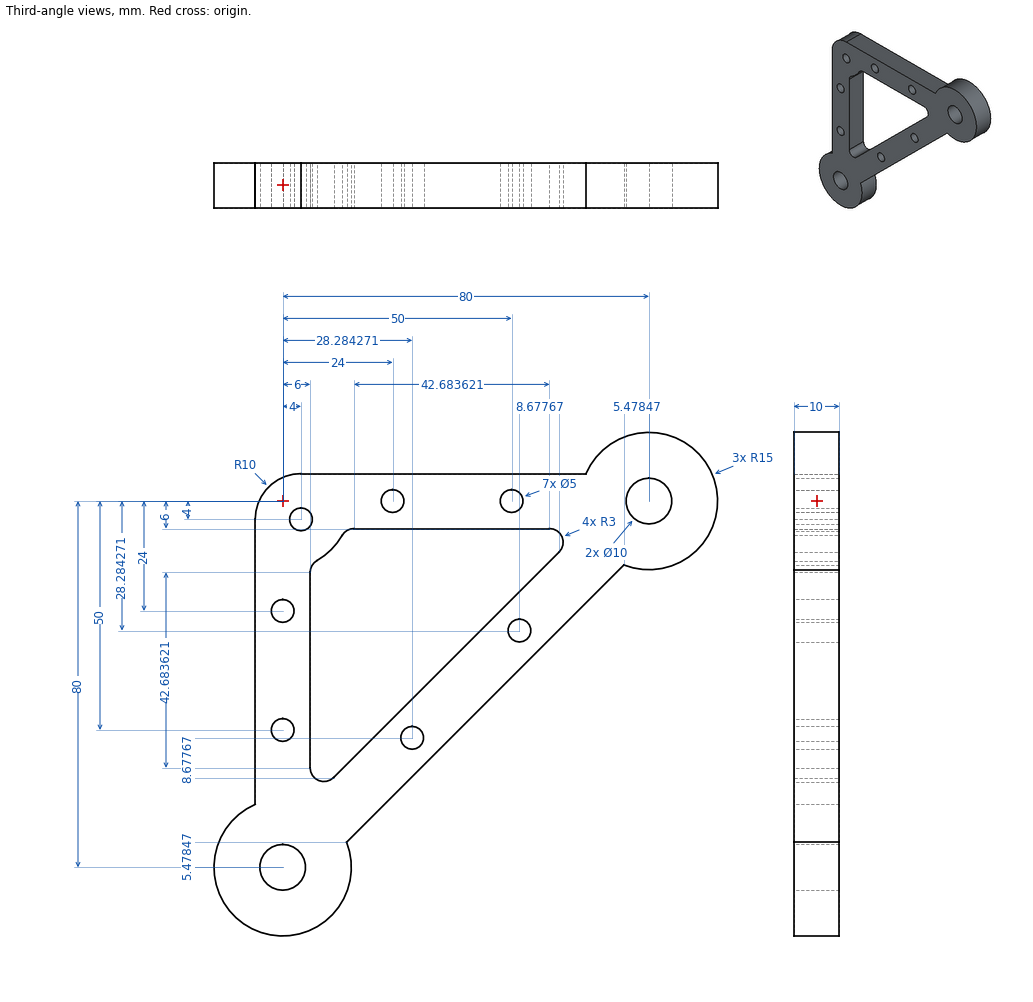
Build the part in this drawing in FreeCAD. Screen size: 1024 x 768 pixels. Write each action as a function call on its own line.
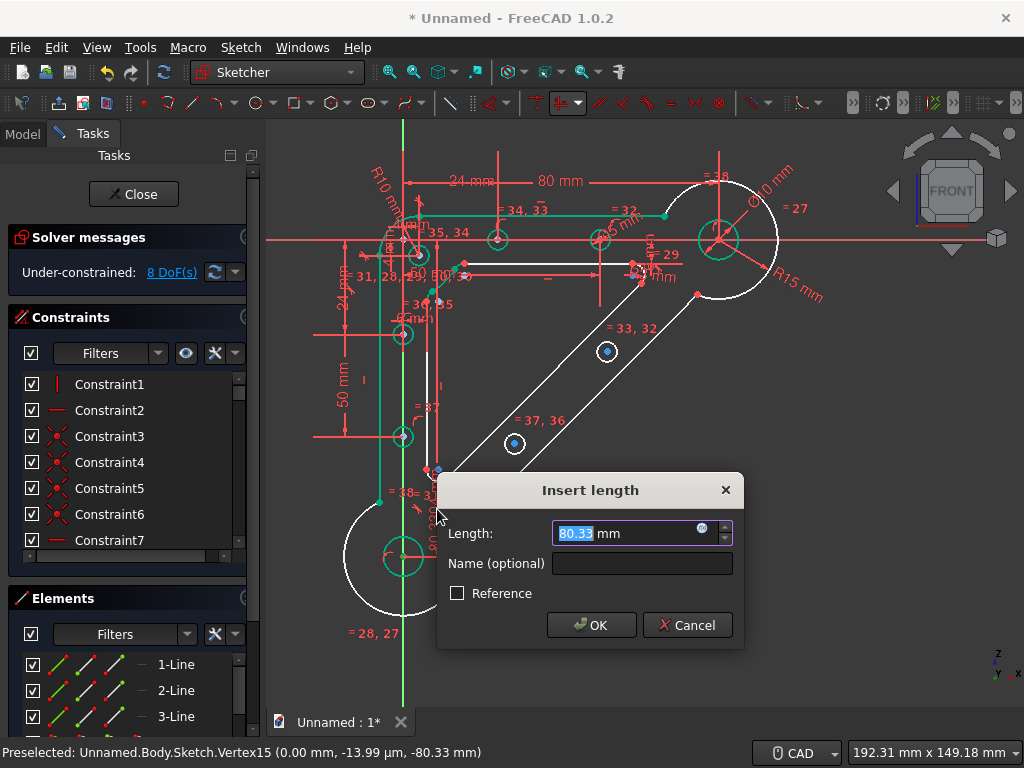
text(80)
key(Return)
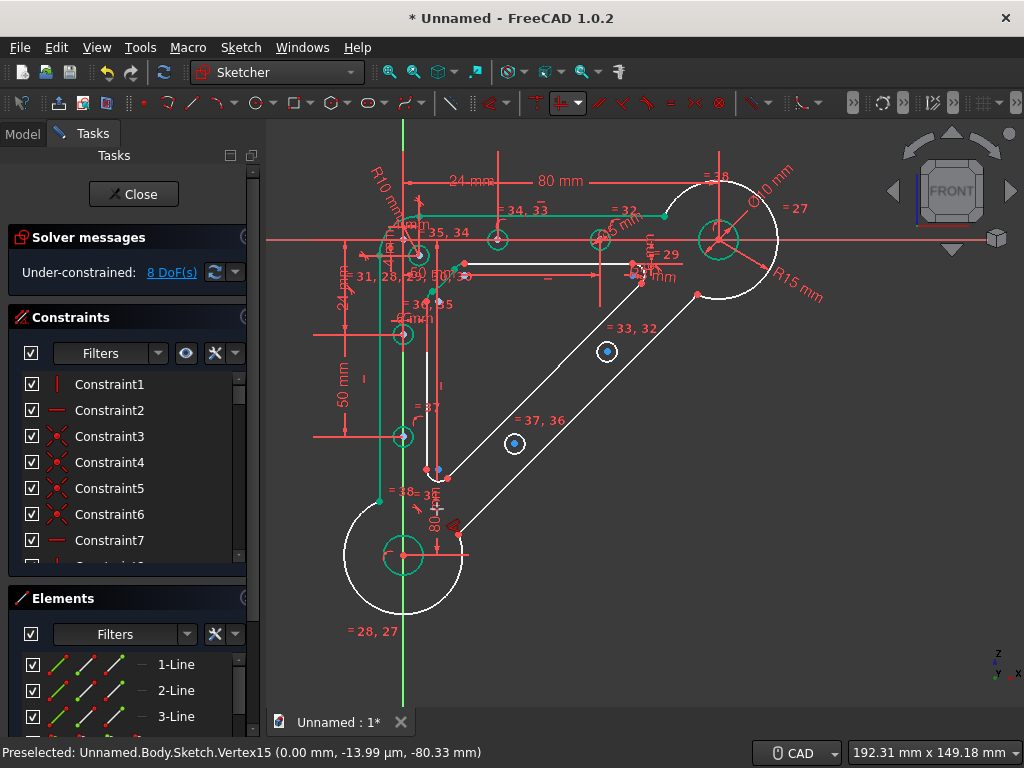
scroll(697, 295, up, 4)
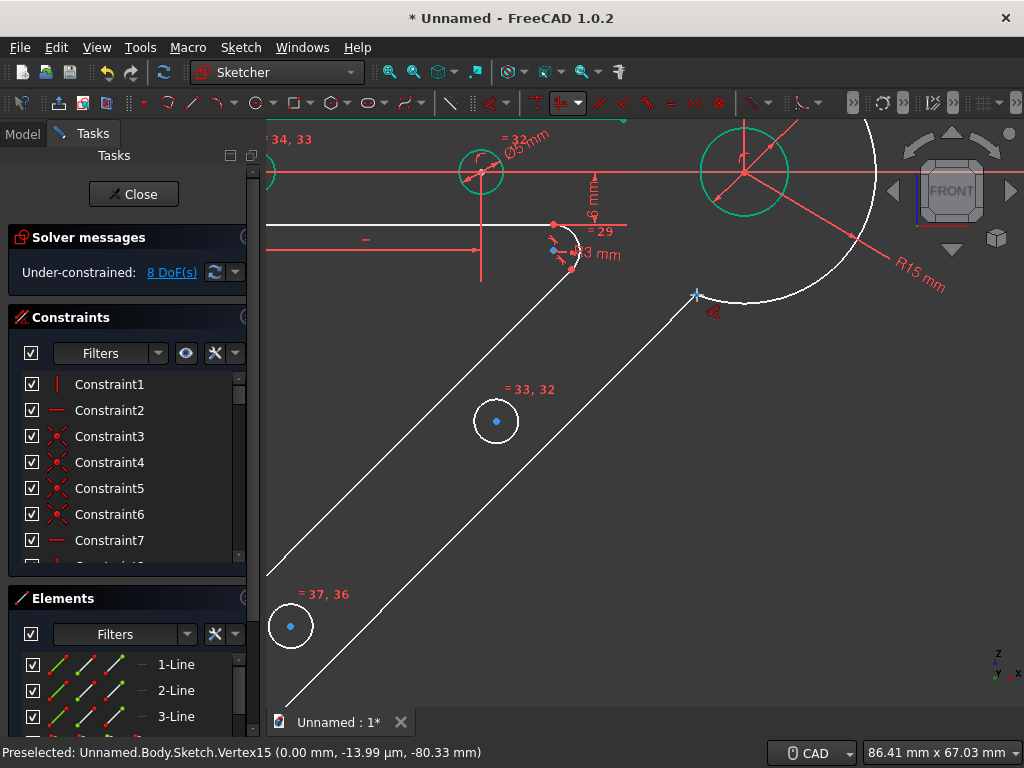
click(696, 295)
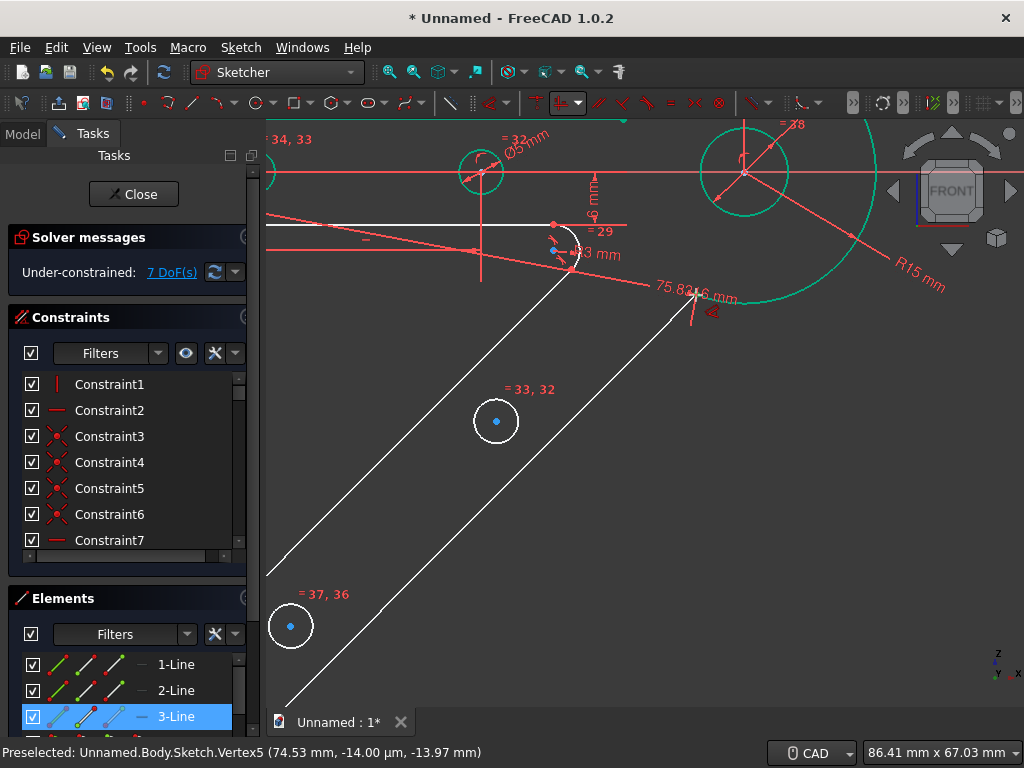
click(744, 172)
click(720, 329)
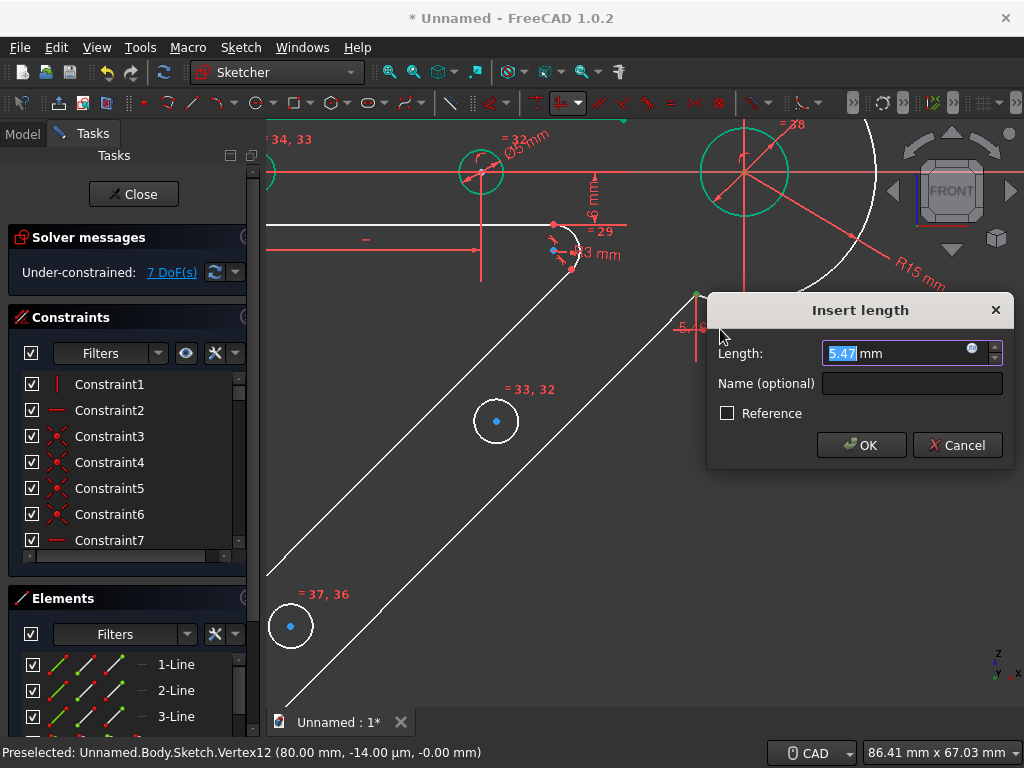
text(5.47847)
key(Return)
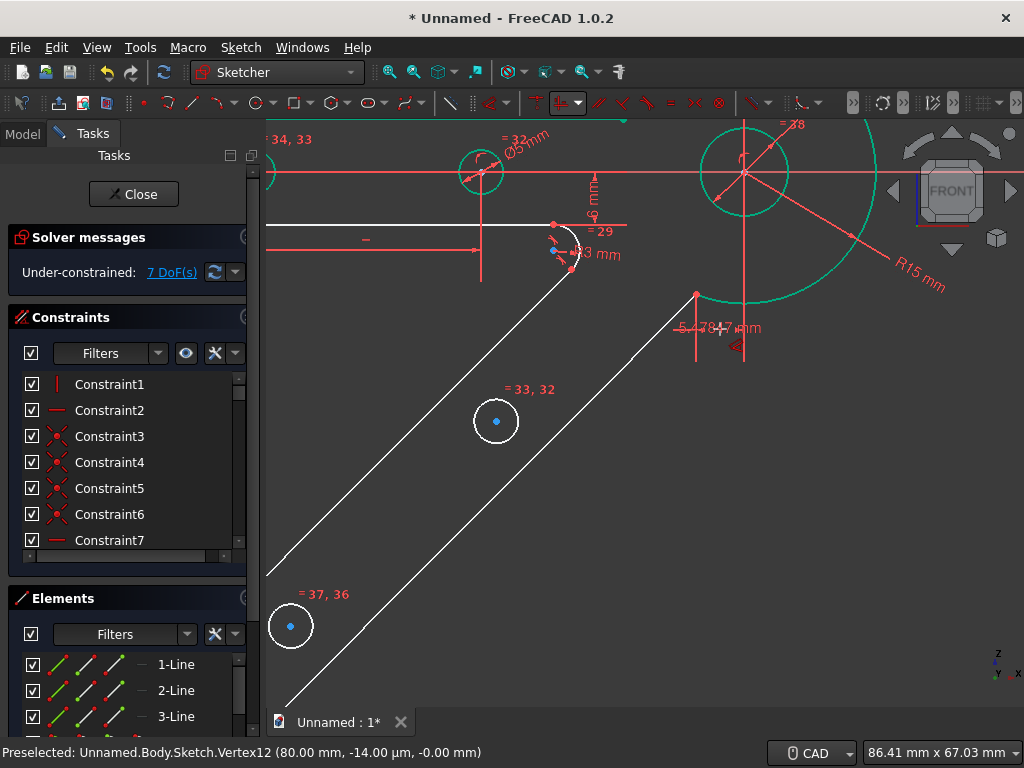
click(572, 270)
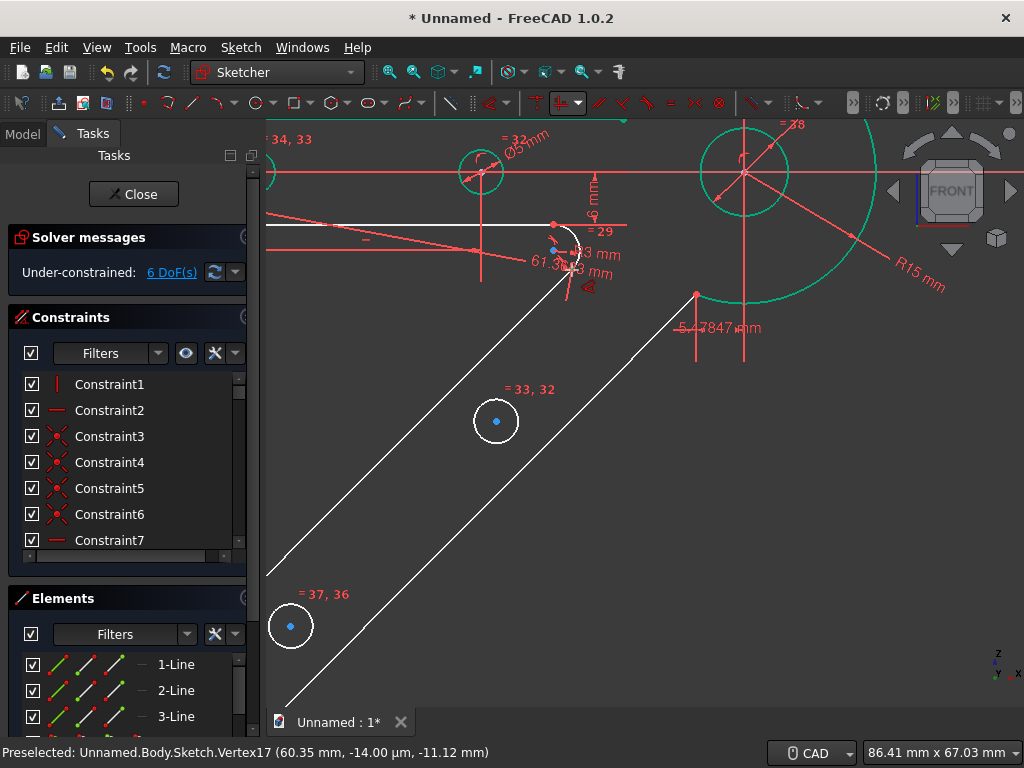
click(496, 421)
click(517, 455)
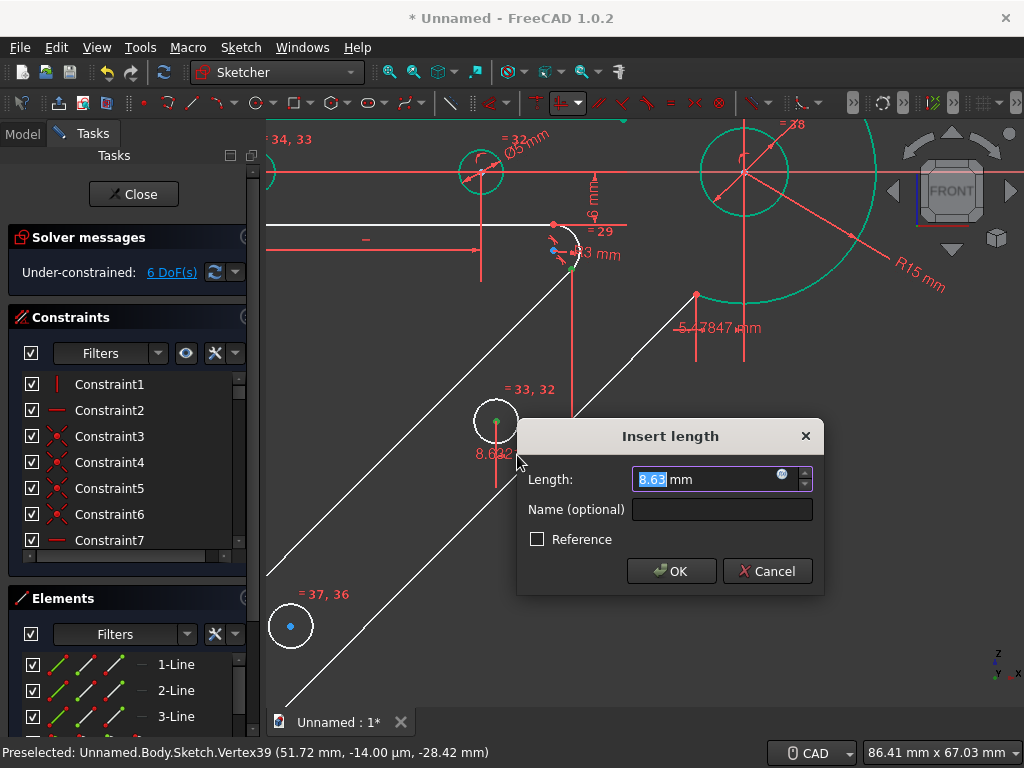
text(8.67767)
key(Return)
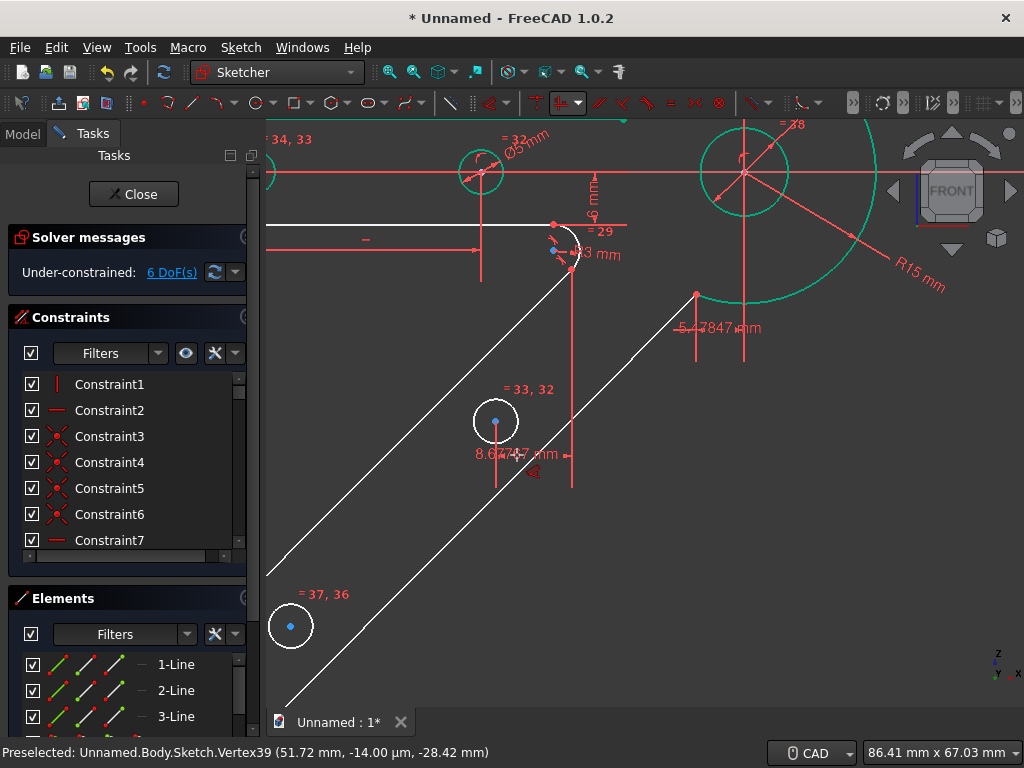
scroll(698, 295, down, 4)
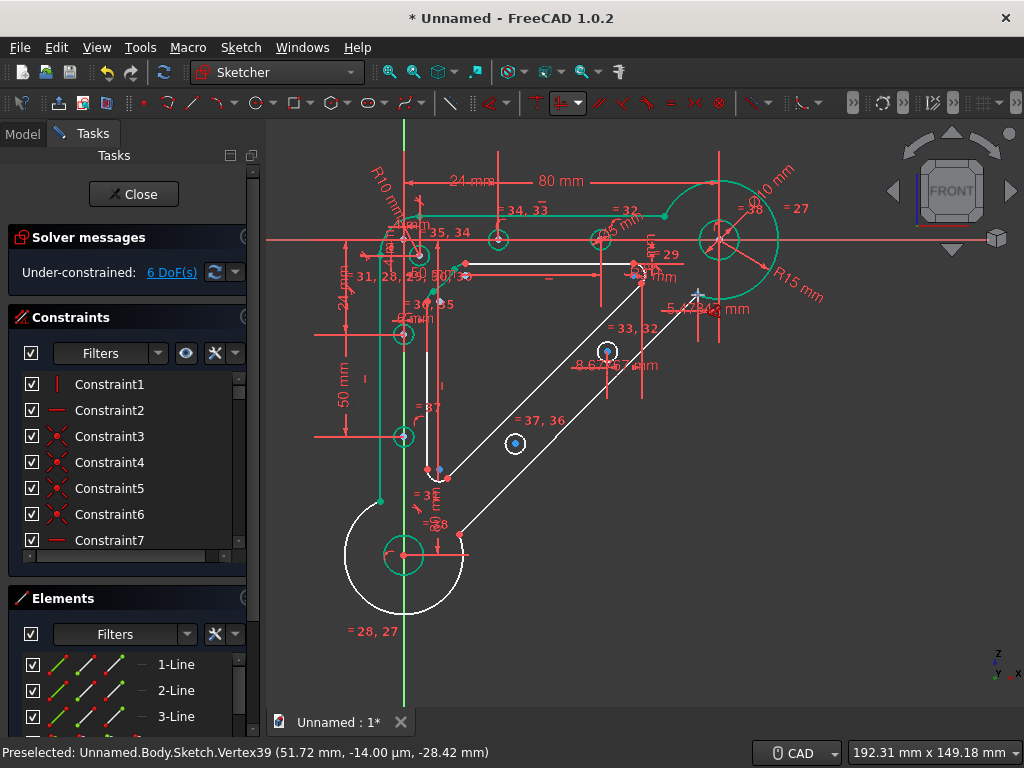
click(448, 478)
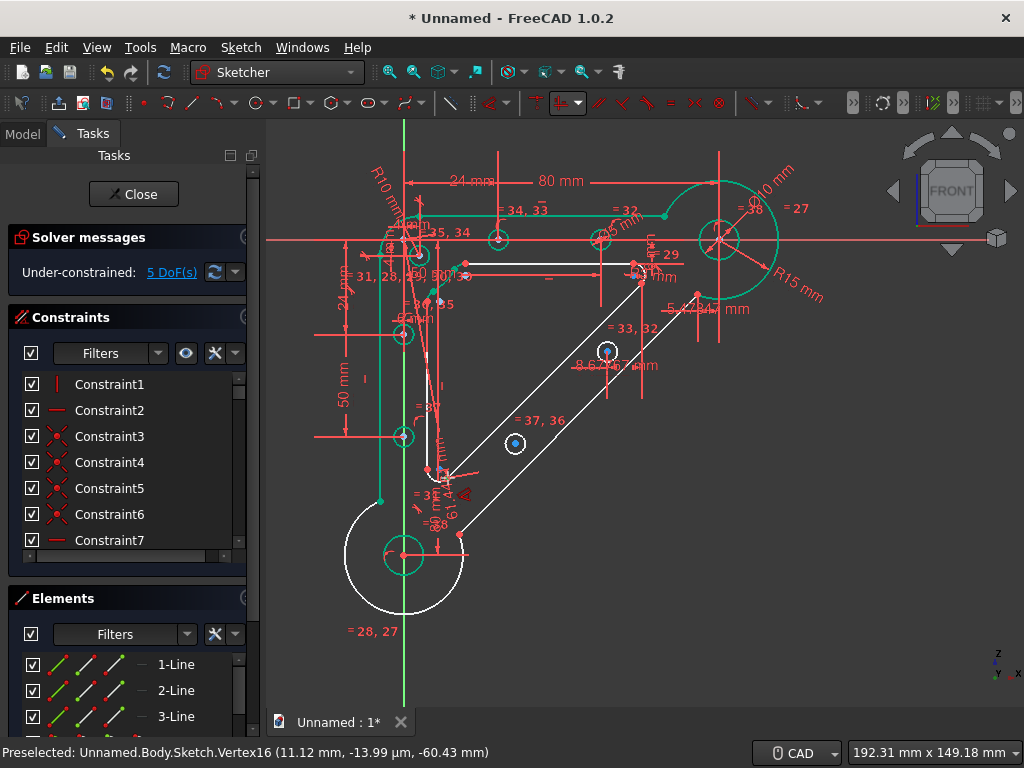
click(515, 444)
click(549, 469)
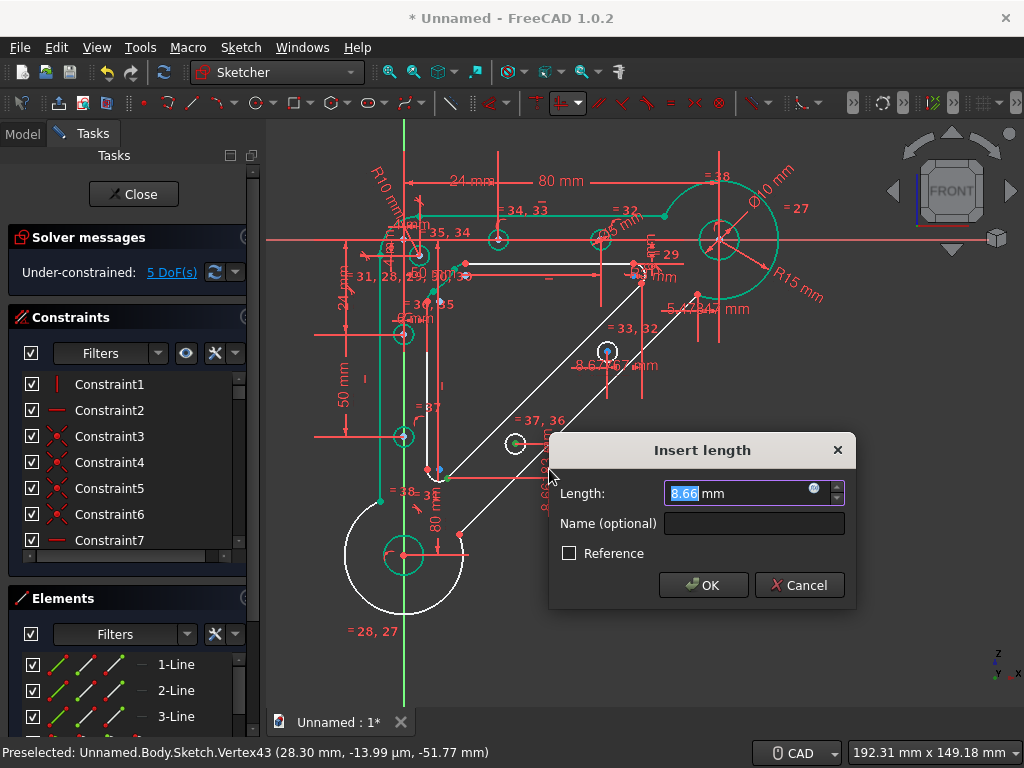
text(8.67767)
key(Return)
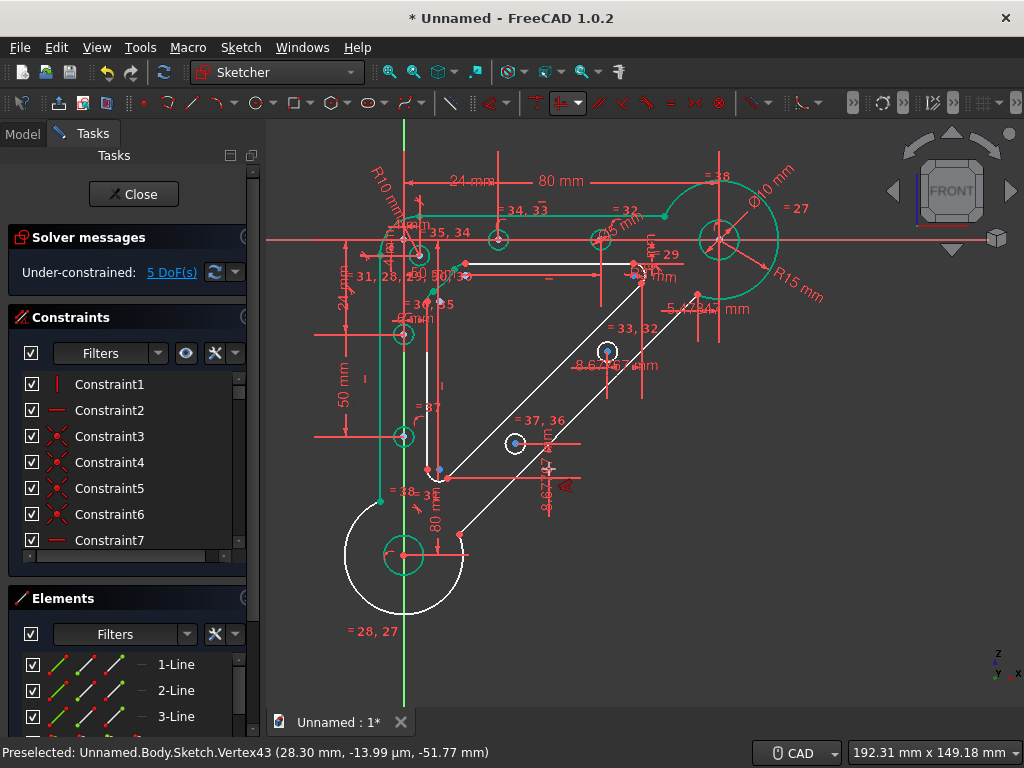
scroll(459, 534, up, 4)